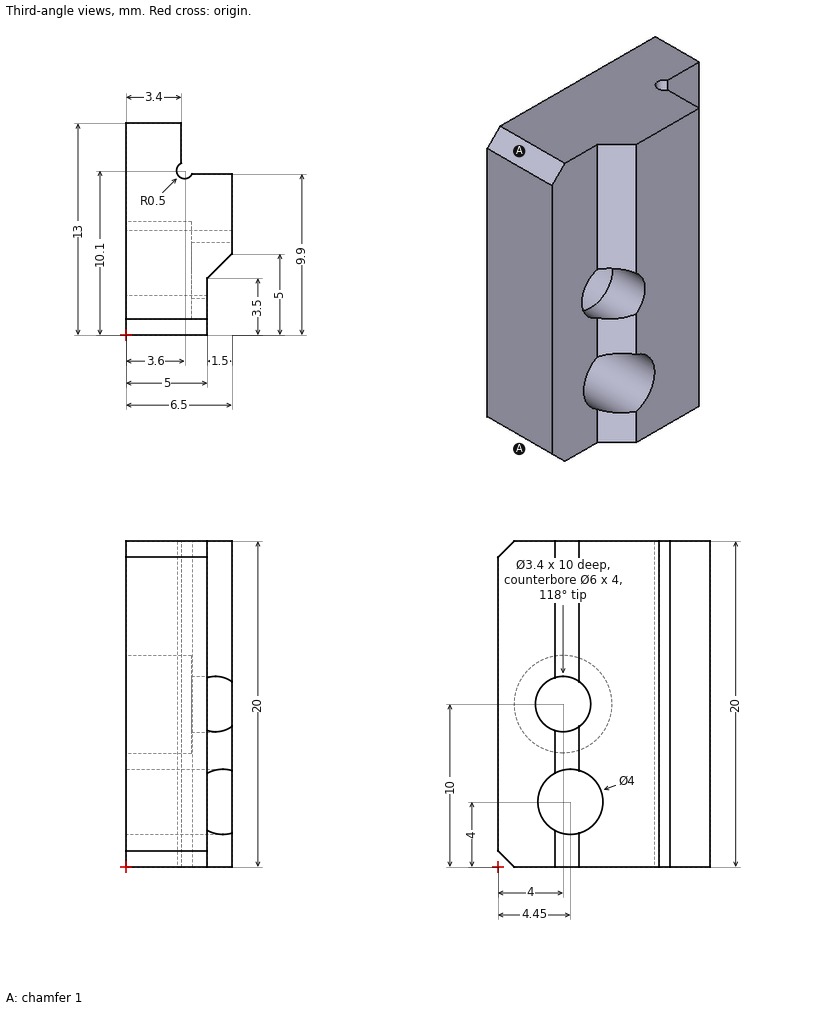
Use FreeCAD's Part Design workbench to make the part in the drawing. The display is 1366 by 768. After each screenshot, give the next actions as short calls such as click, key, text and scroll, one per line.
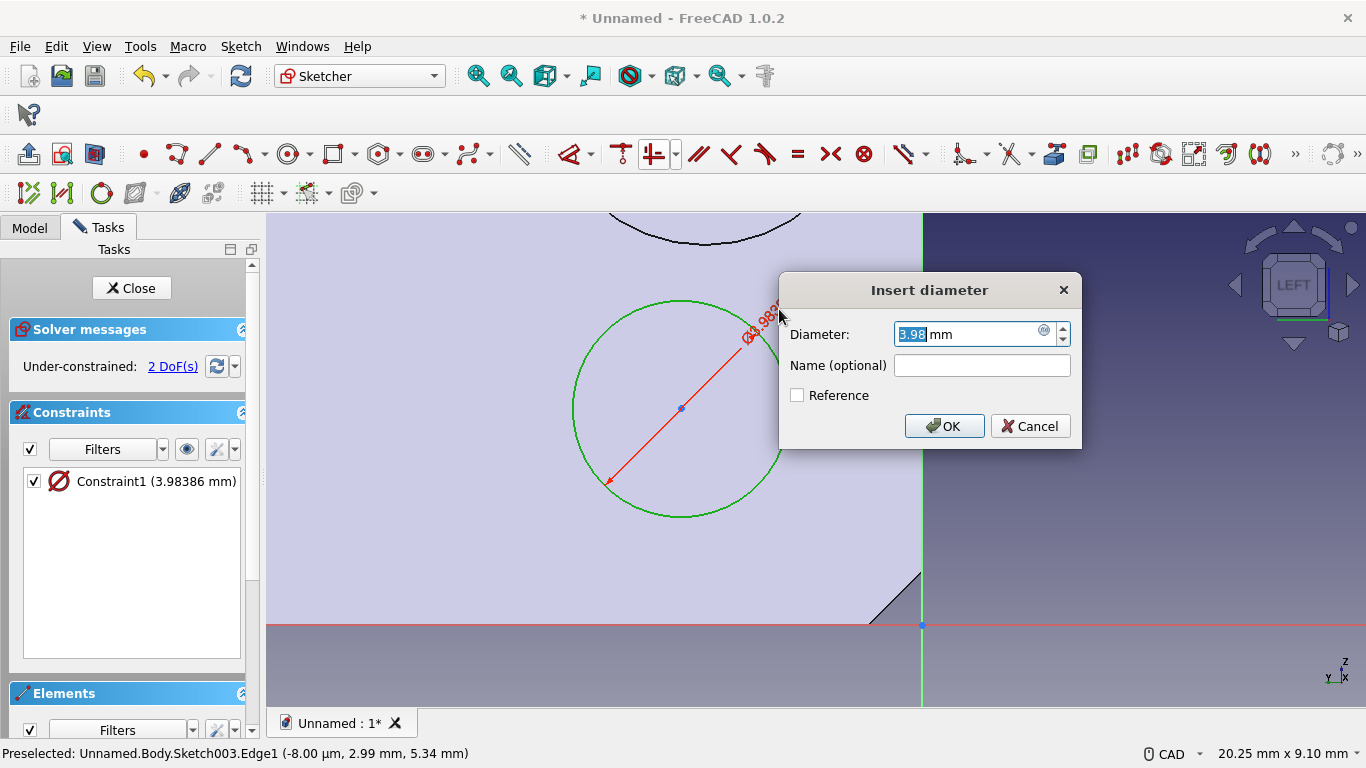
text(4)
key(Return)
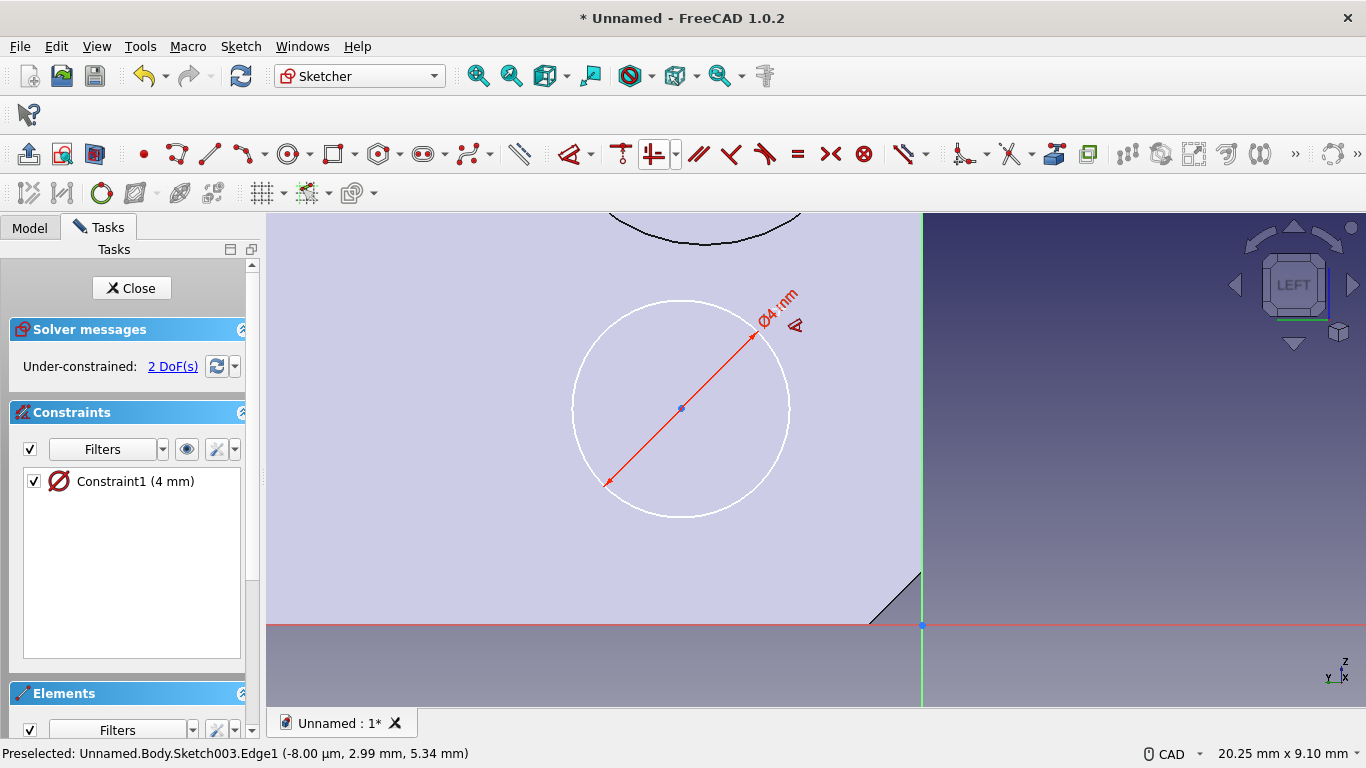
click(681, 409)
click(956, 517)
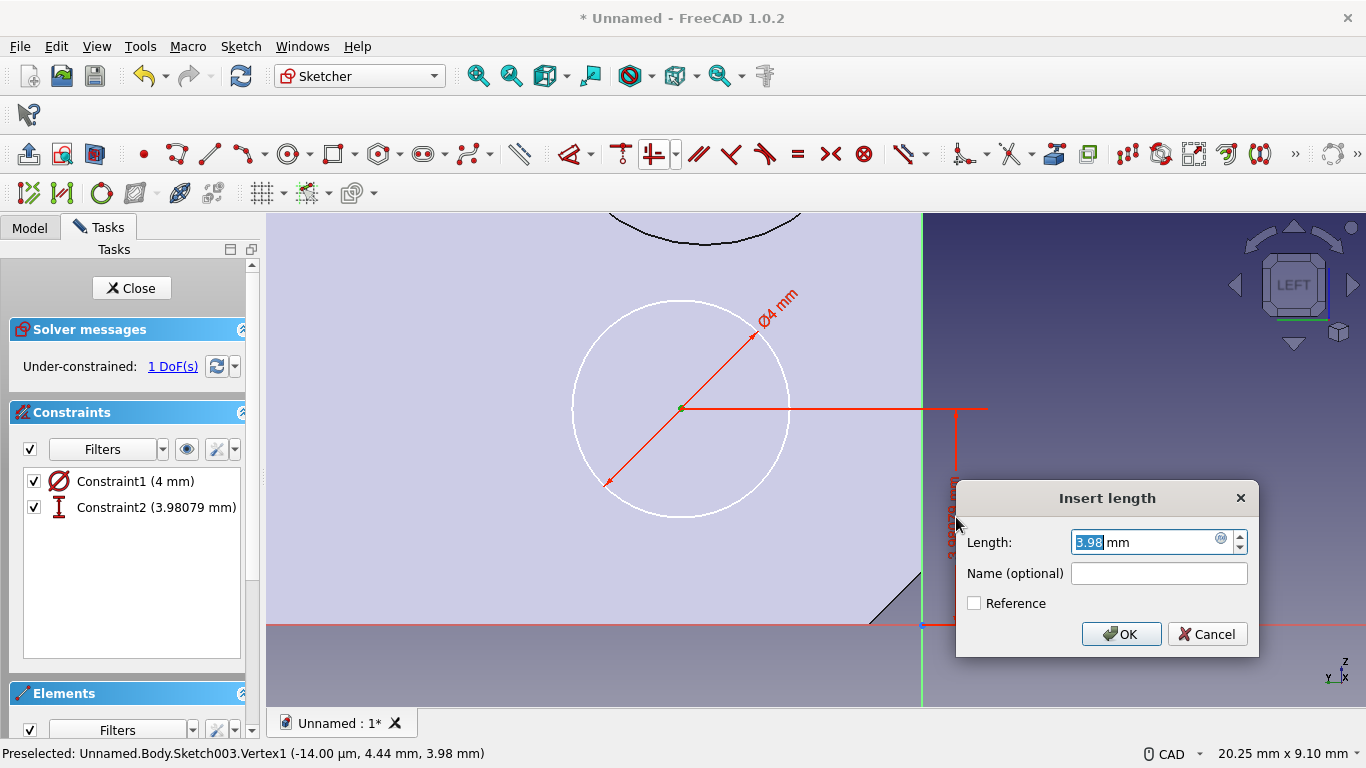
text(4)
key(Return)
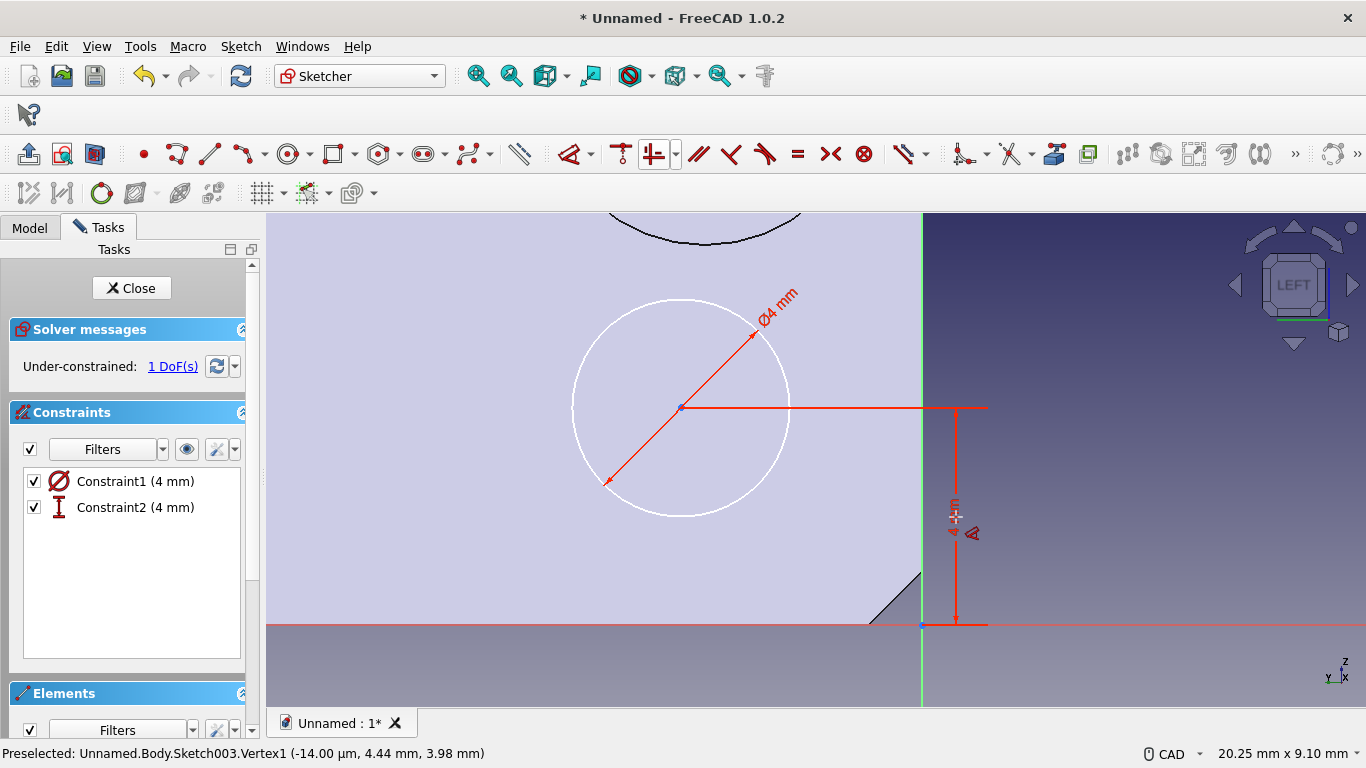
click(681, 408)
click(802, 659)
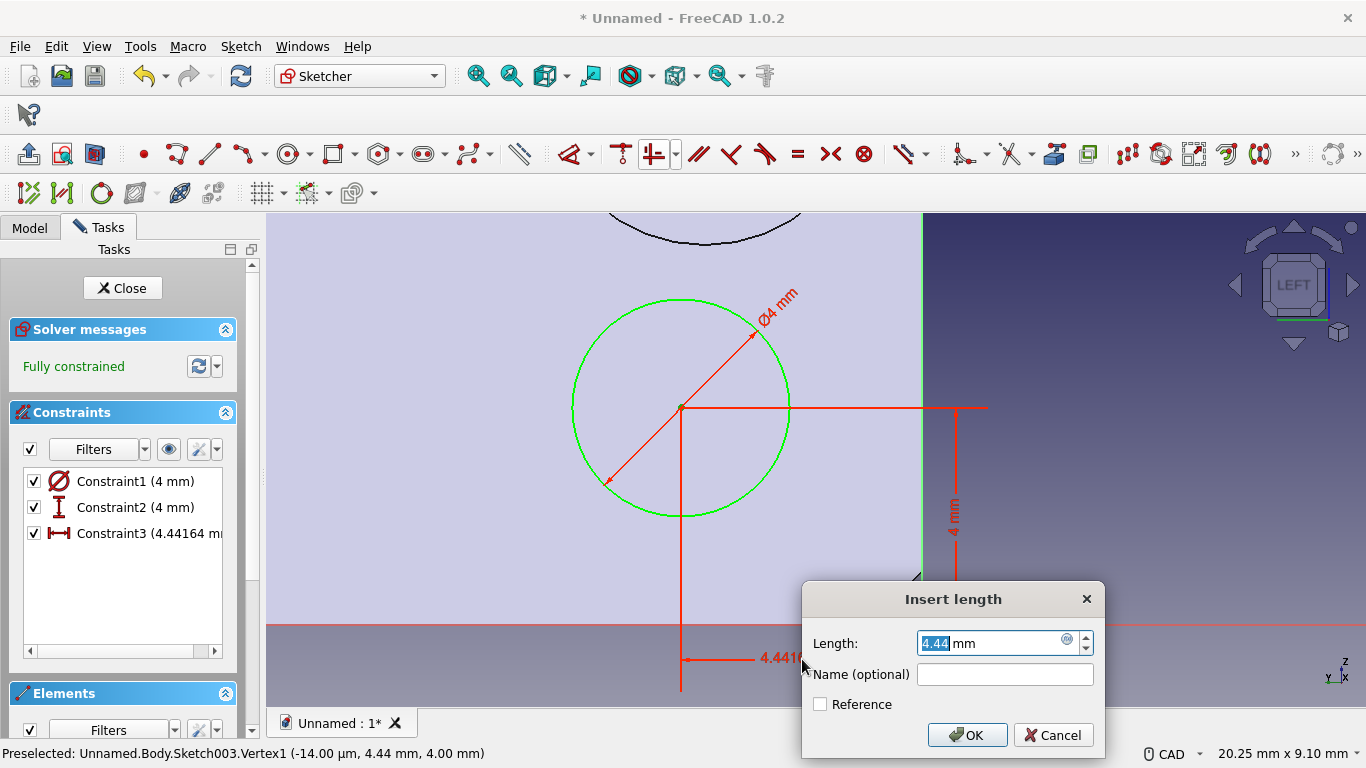
text(4.45)
key(Return)
key(Escape)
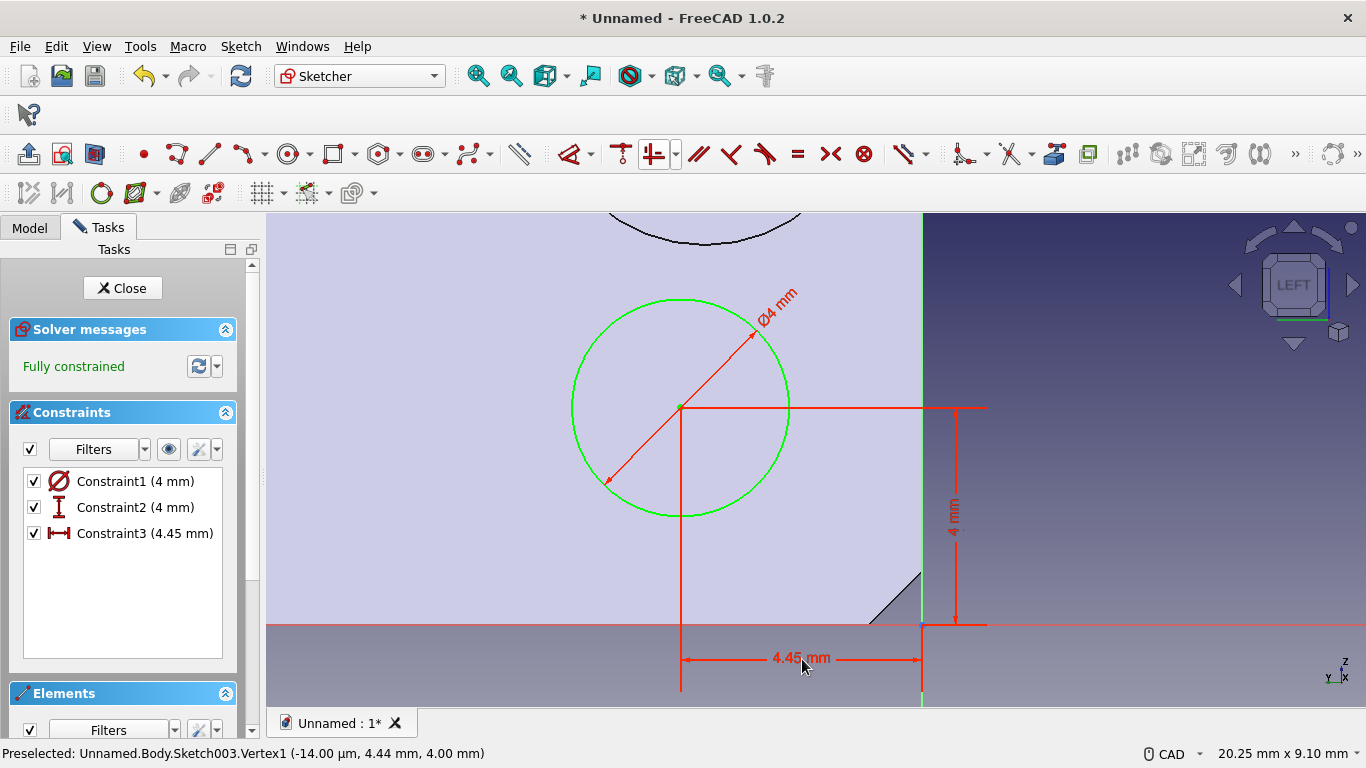
click(123, 288)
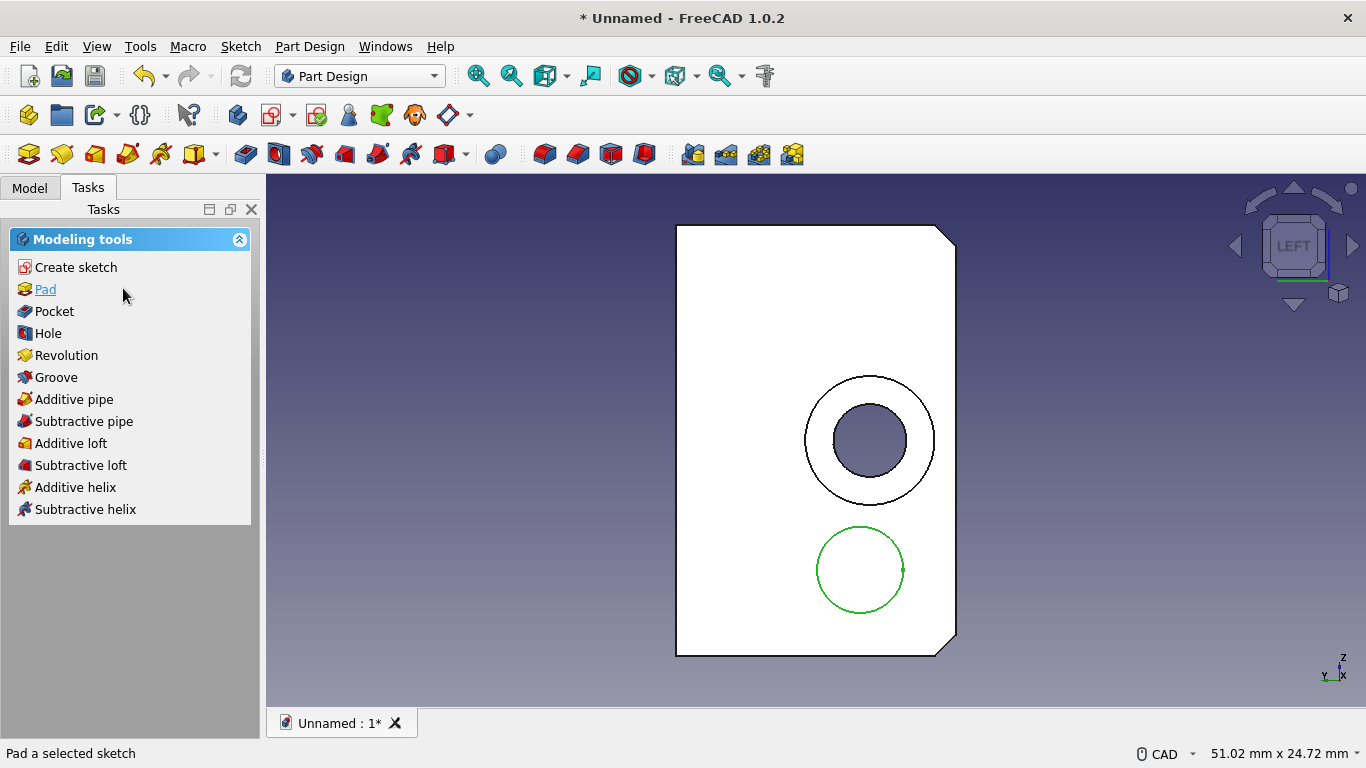
click(246, 154)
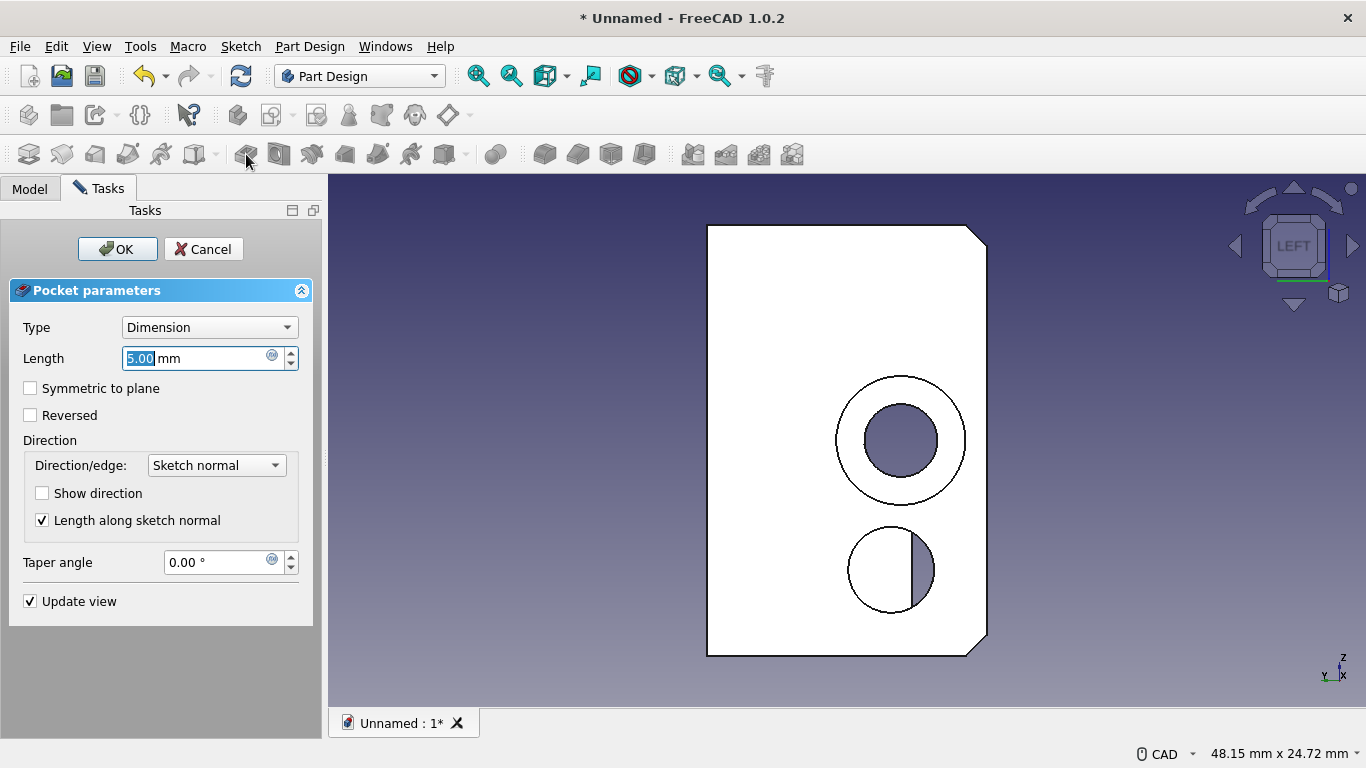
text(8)
key(Tab)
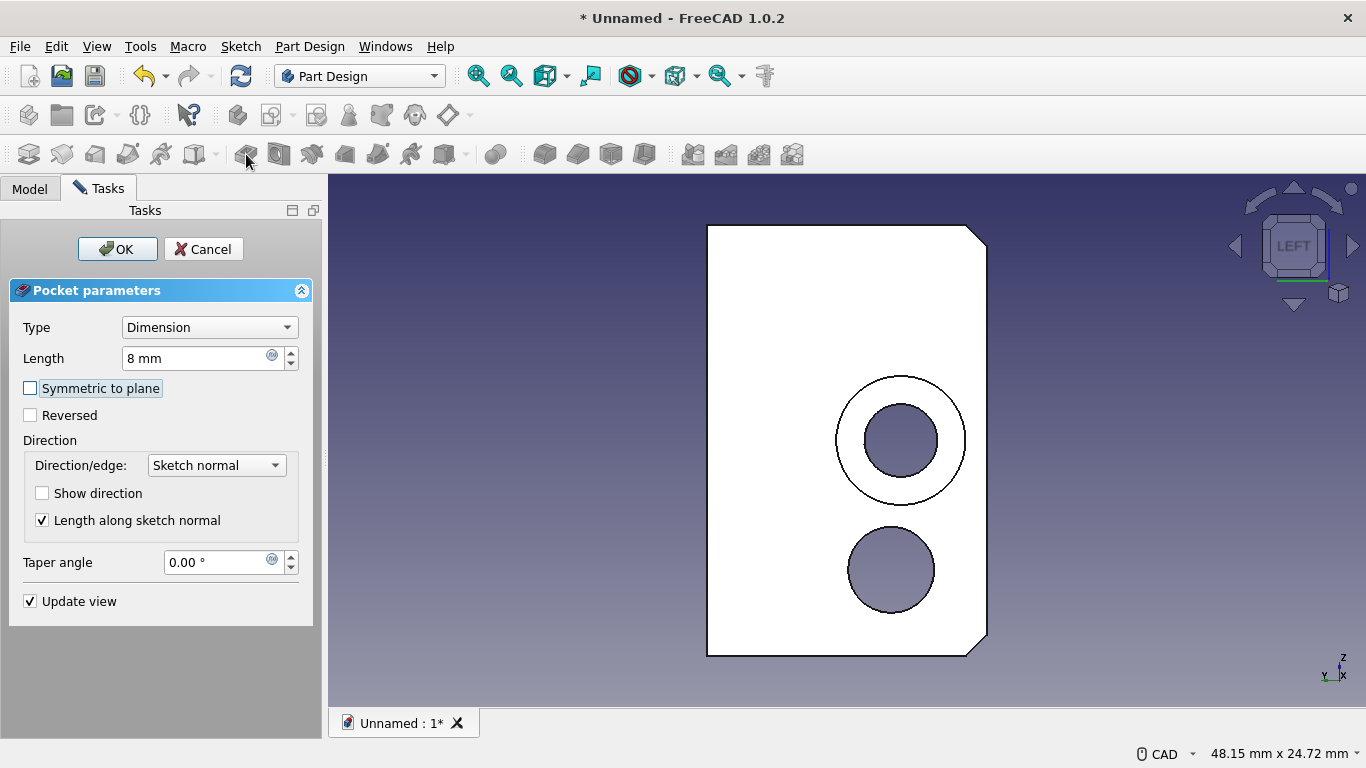
click(118, 249)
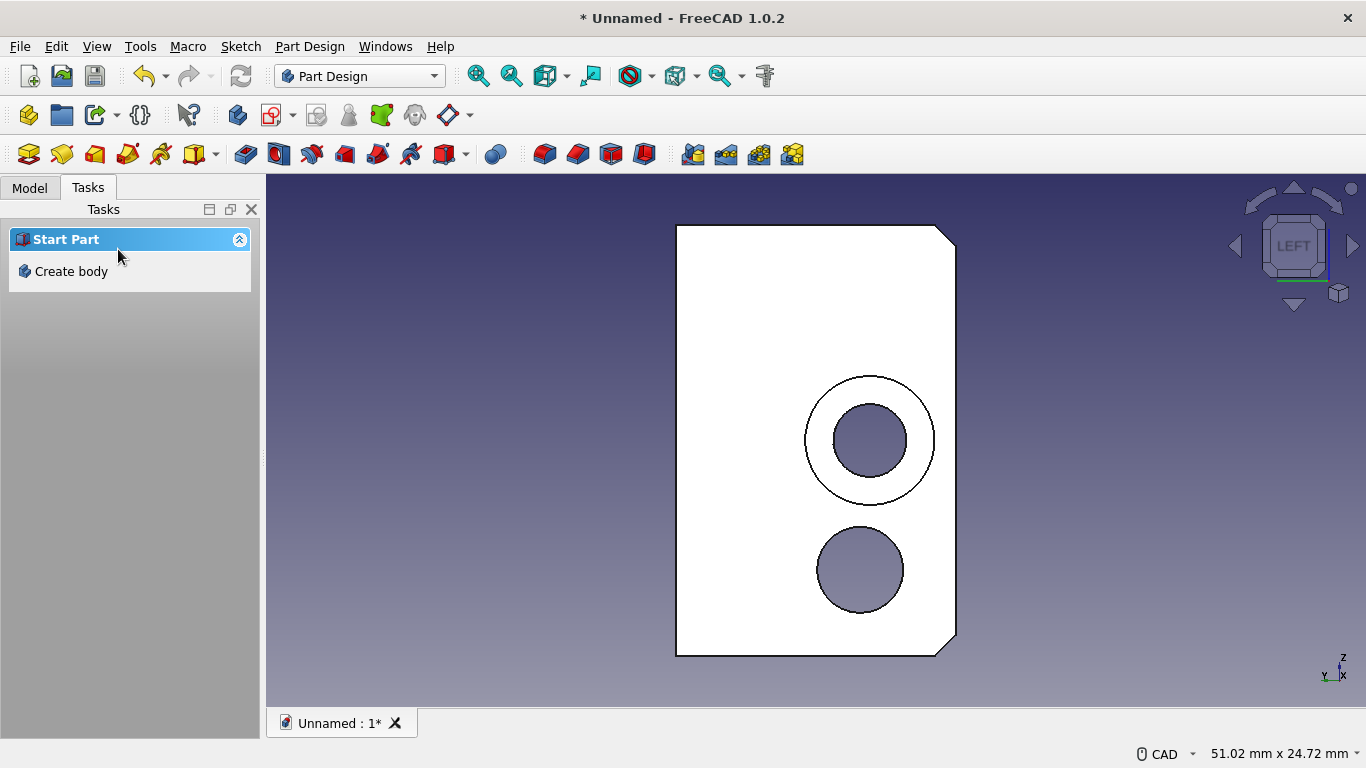
key(0)